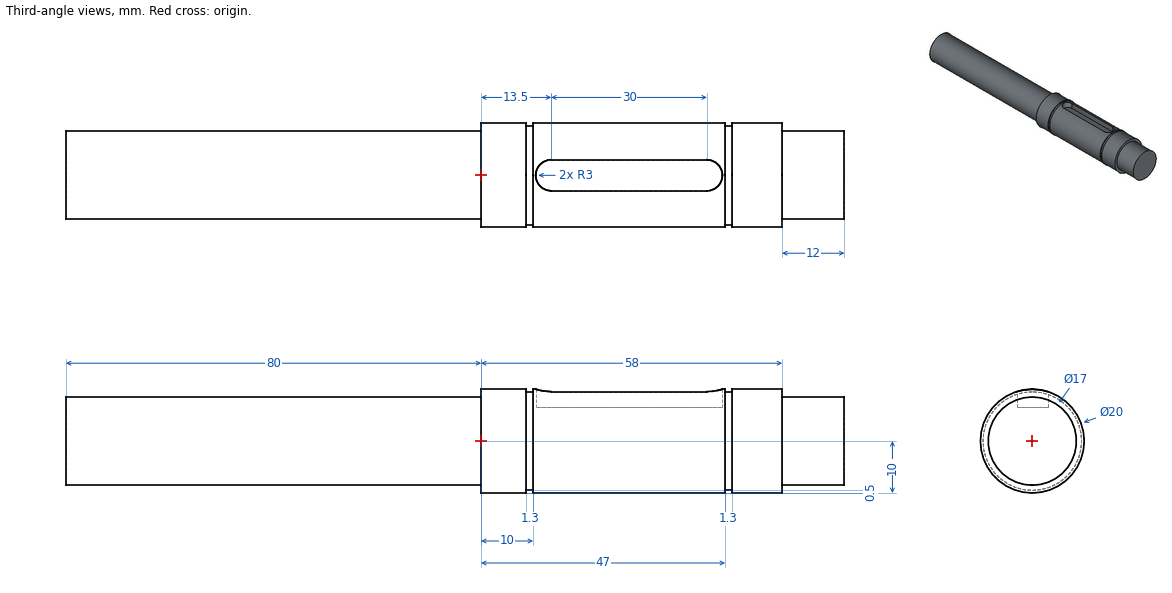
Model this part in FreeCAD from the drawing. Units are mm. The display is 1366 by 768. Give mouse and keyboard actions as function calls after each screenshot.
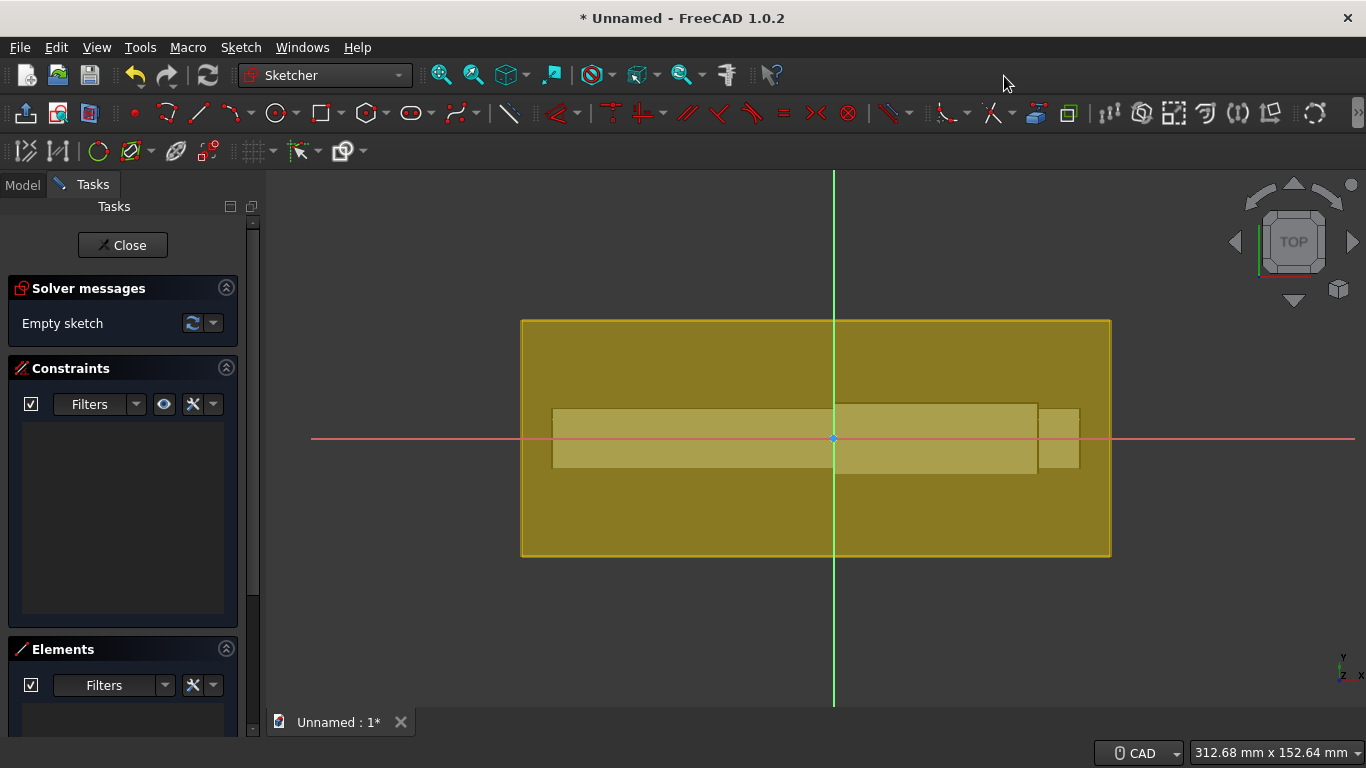
scroll(970, 438, up, 7)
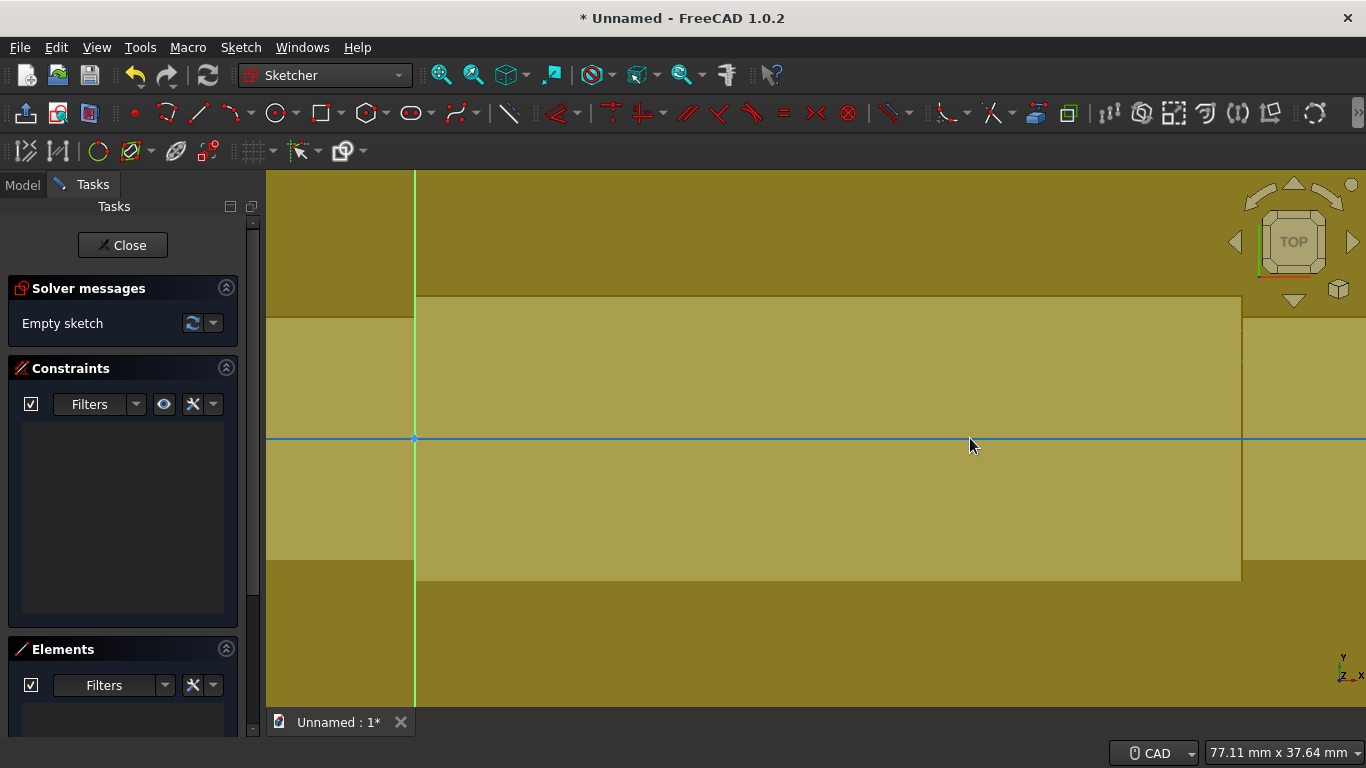
key(g)
key(s)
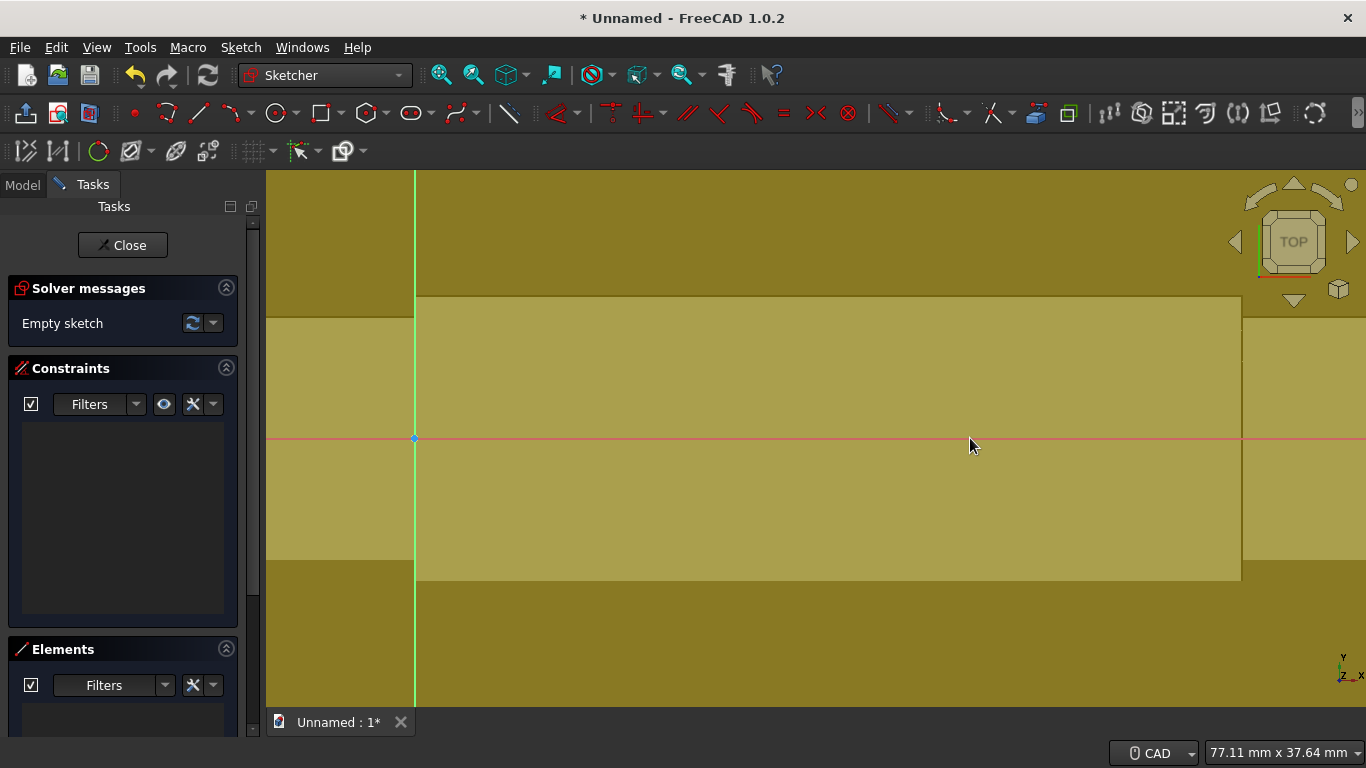
click(607, 438)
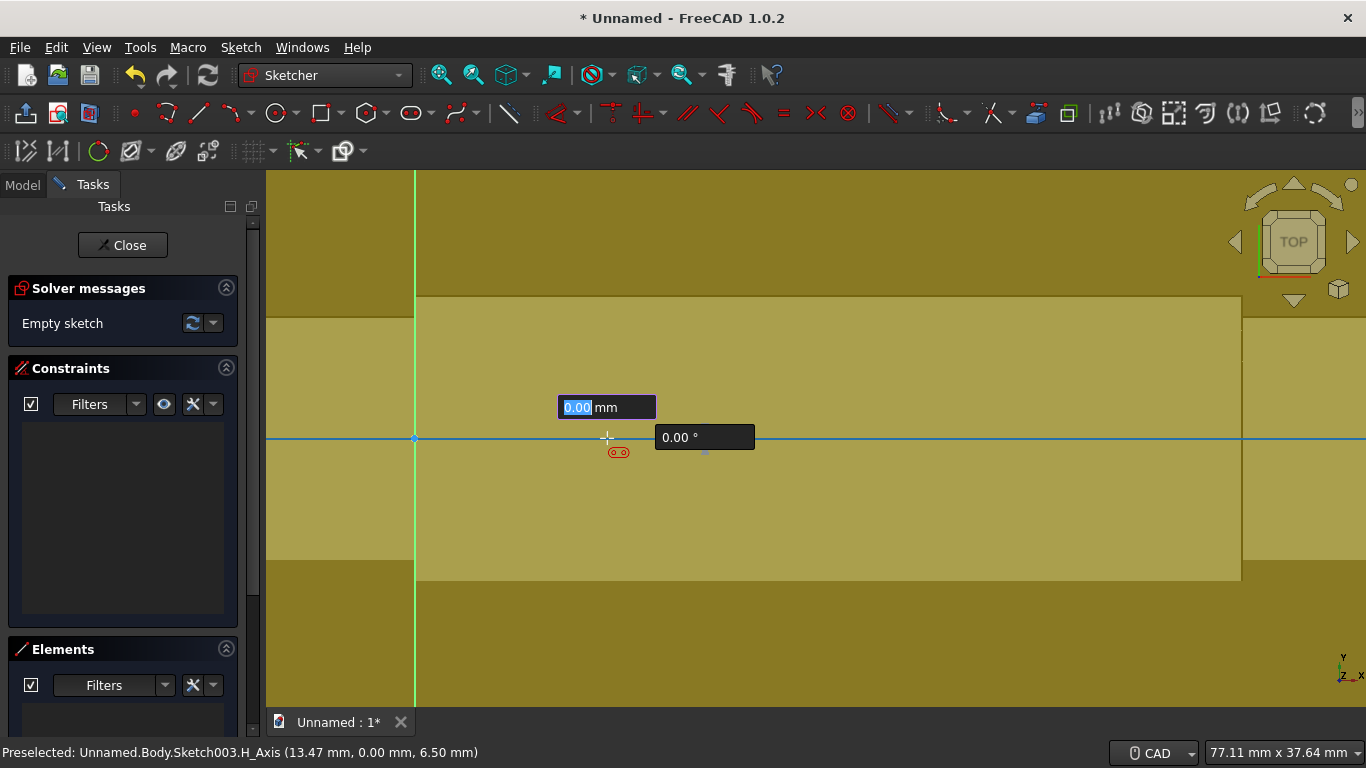
click(1035, 430)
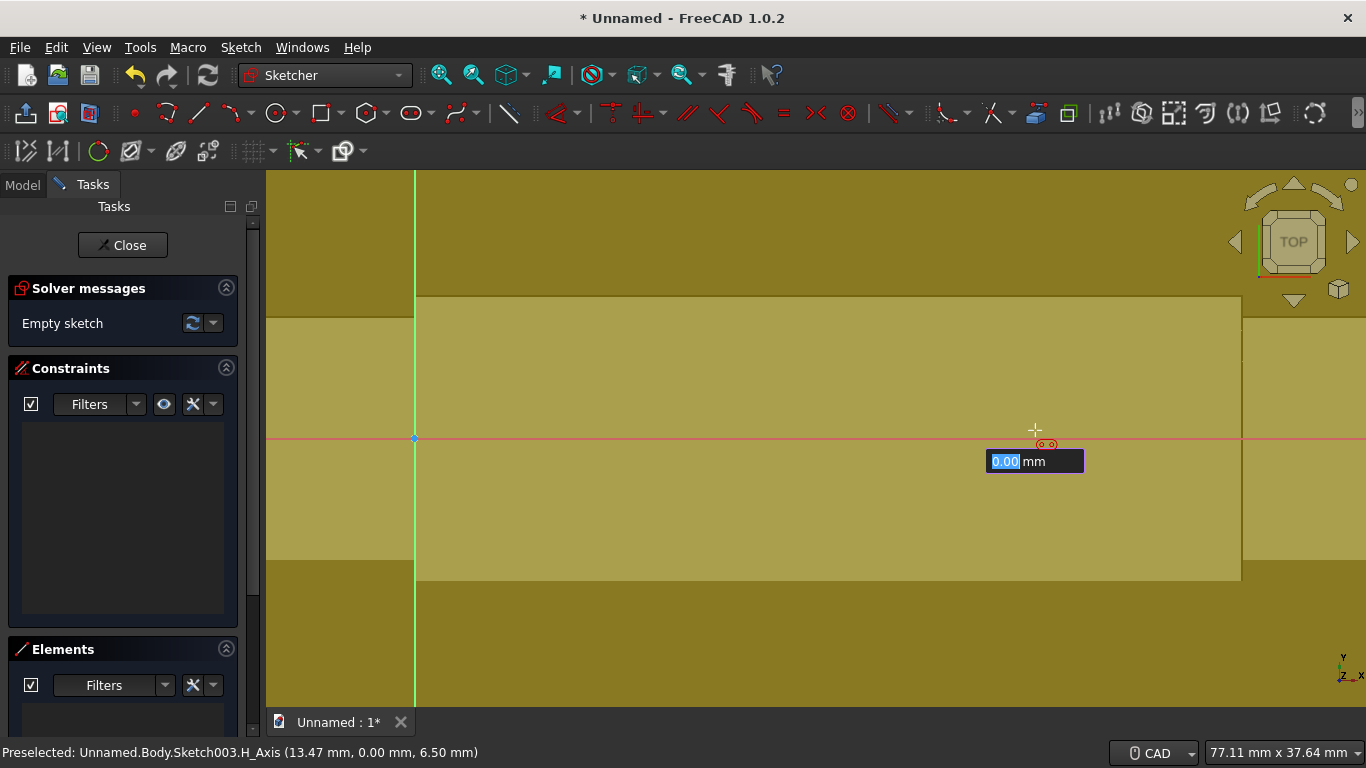
click(821, 396)
key(Escape)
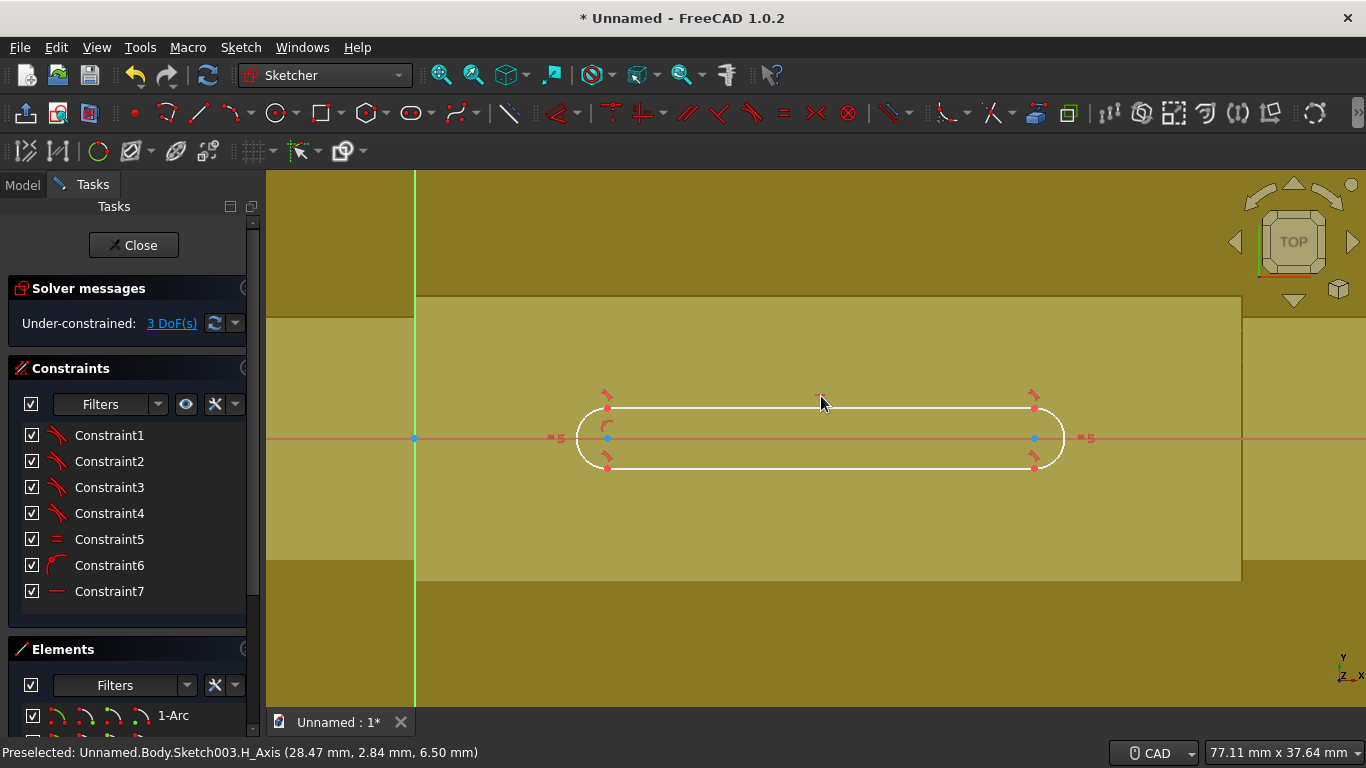
key(d)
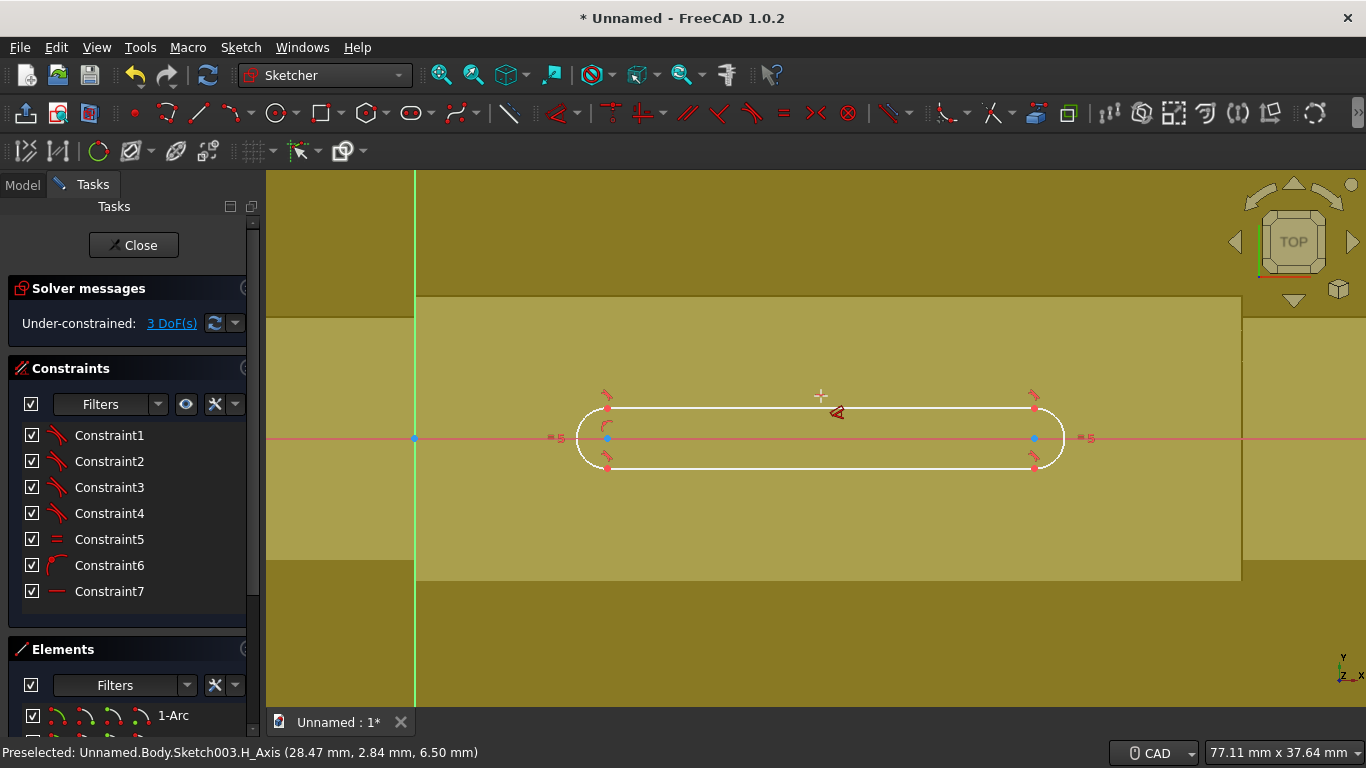
click(583, 421)
click(557, 402)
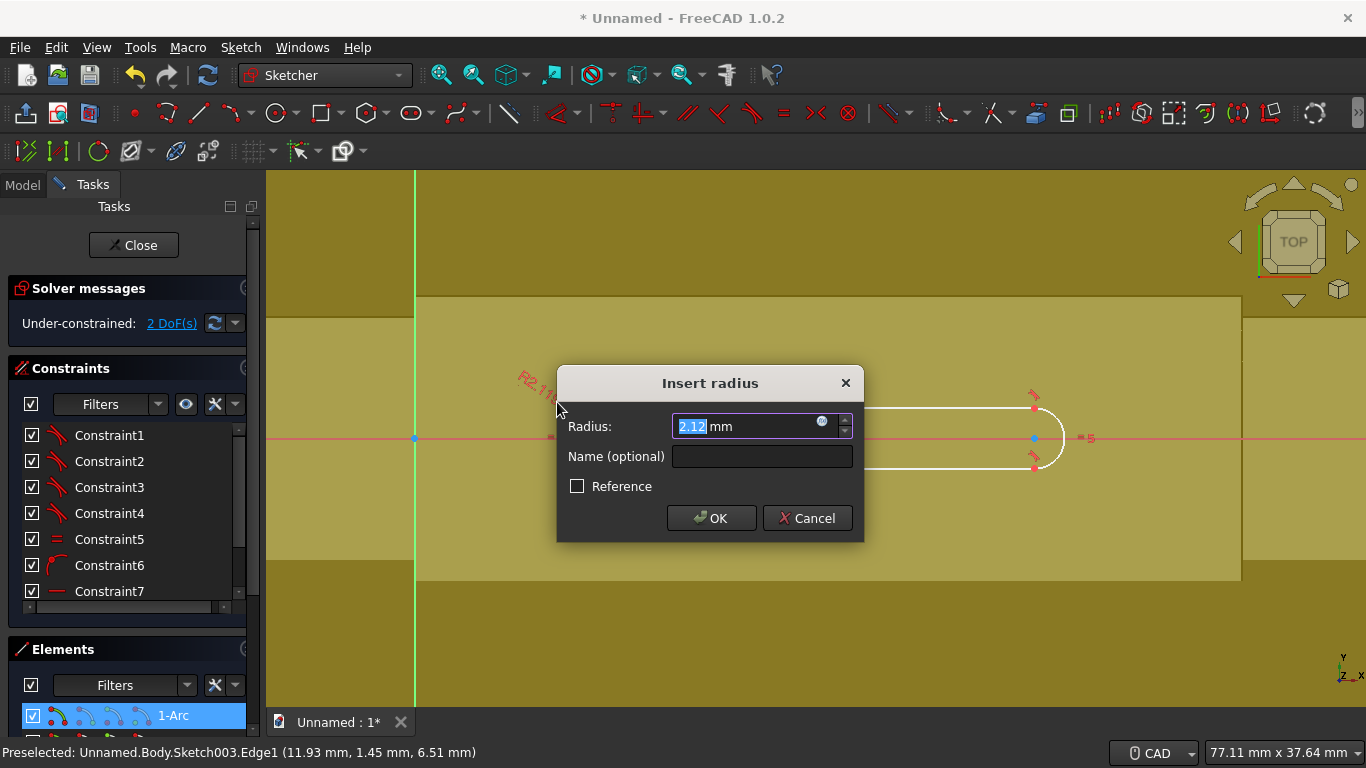
text(3)
key(Return)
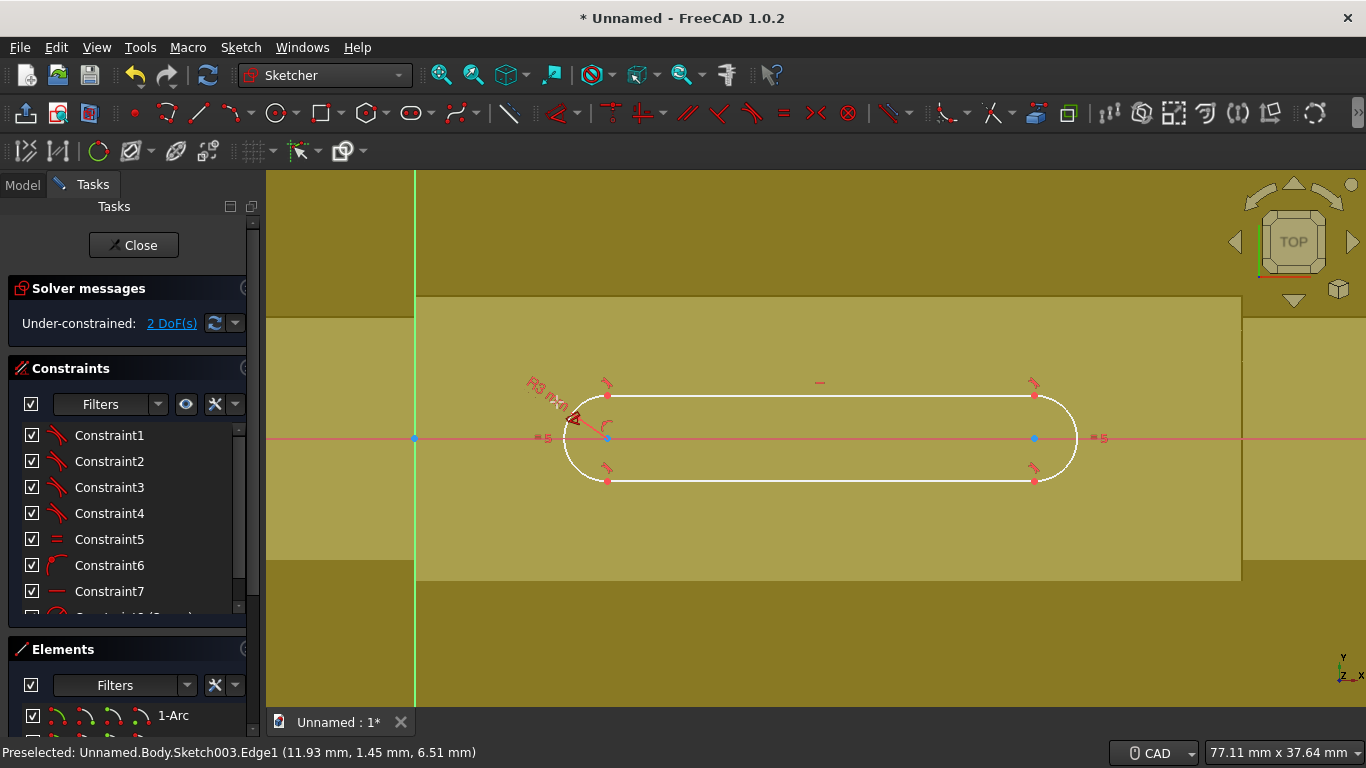
click(735, 396)
click(821, 362)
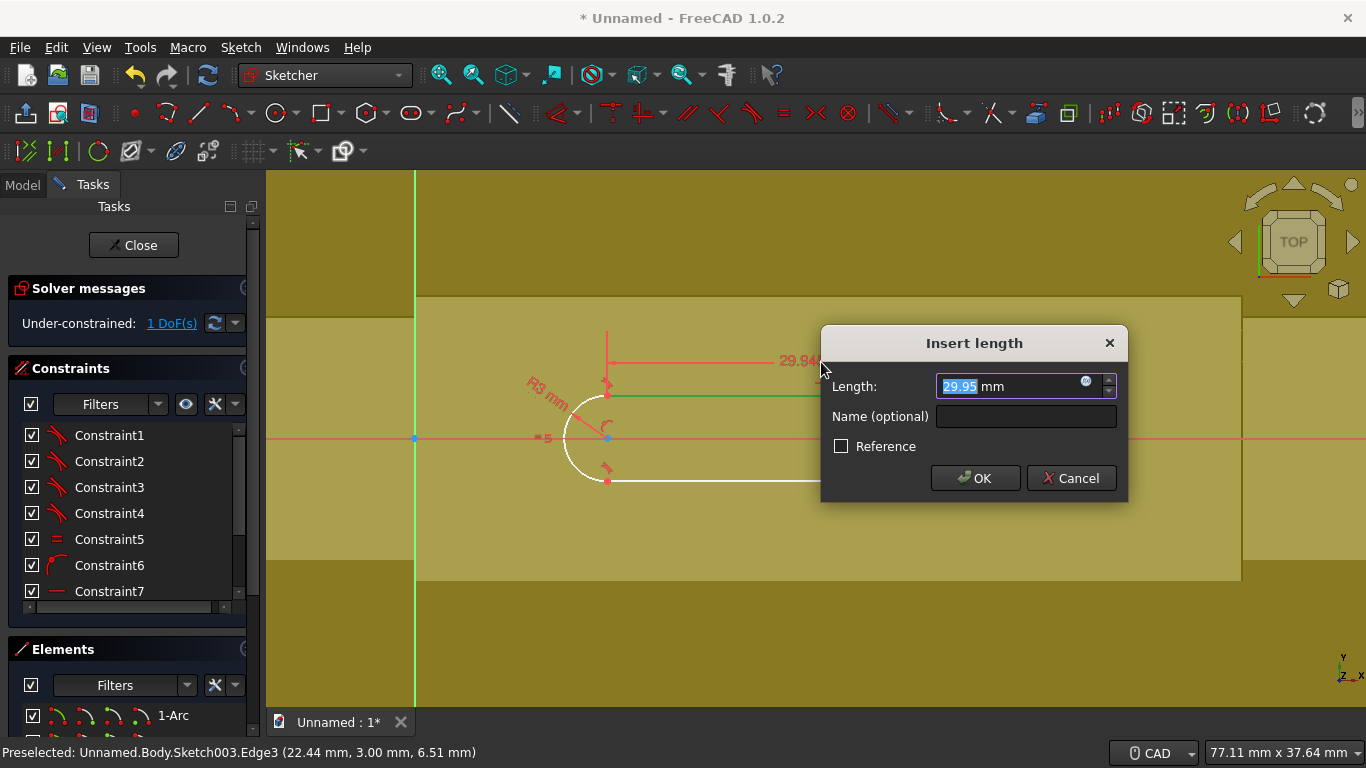
text(30)
key(Return)